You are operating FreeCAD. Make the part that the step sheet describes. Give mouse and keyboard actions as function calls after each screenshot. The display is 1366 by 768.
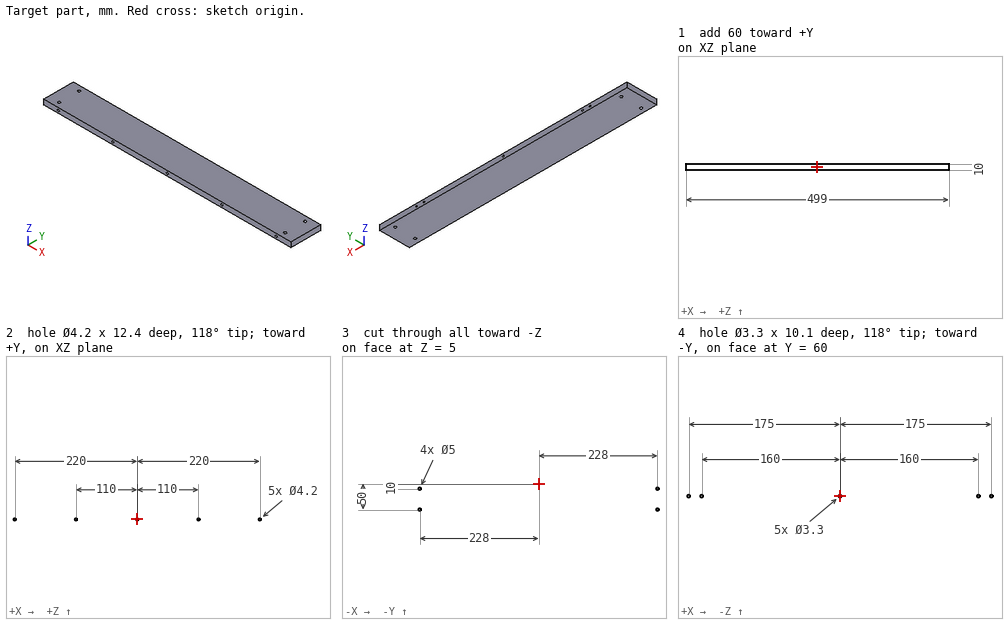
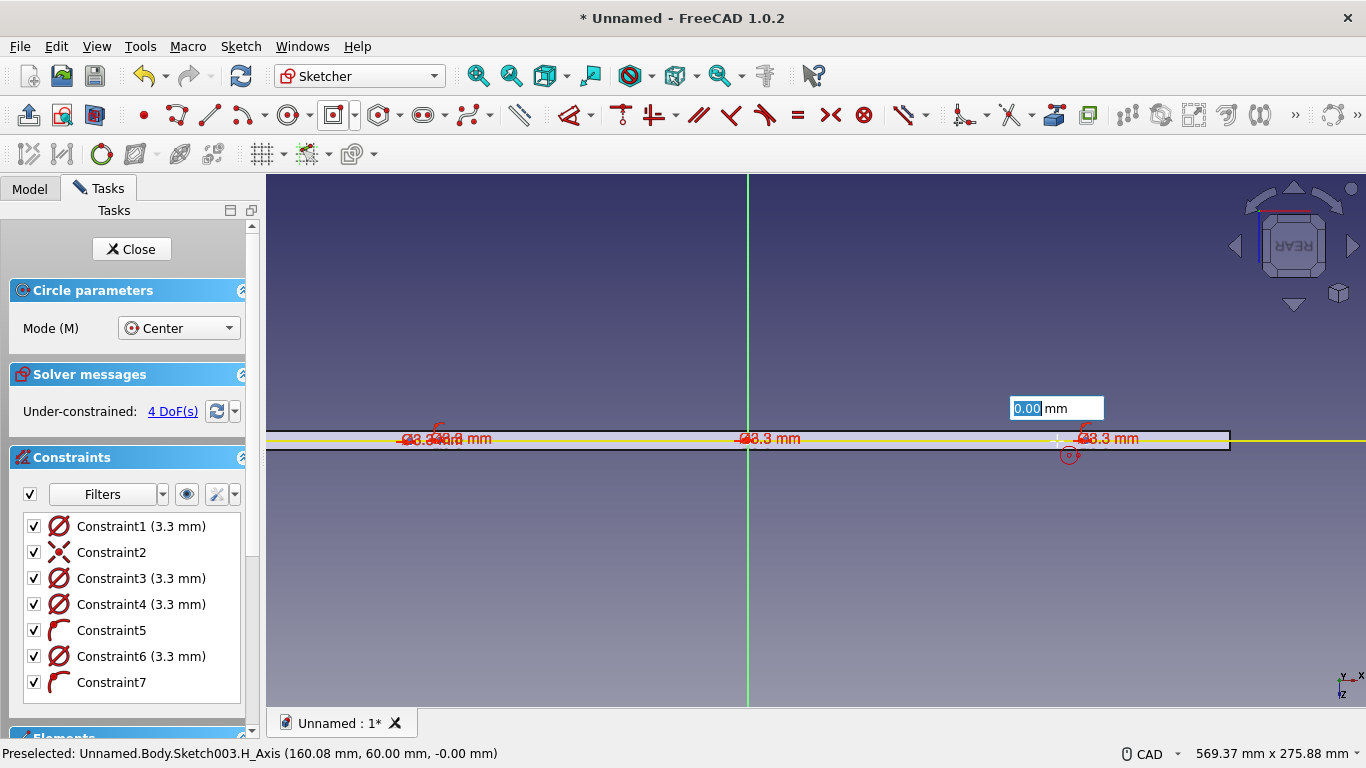
scroll(1056, 444, up, 9)
move(1051, 439)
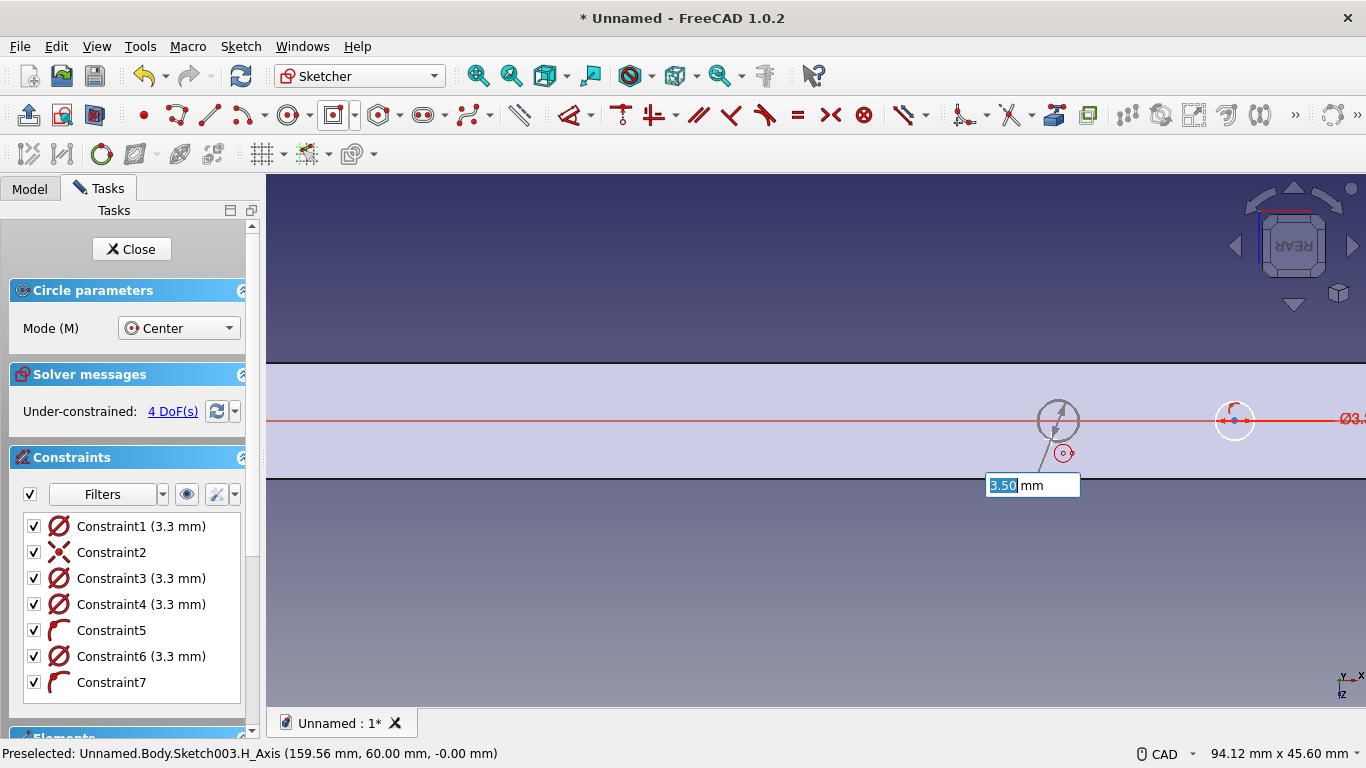
text(3.3)
key(Return)
key(Escape)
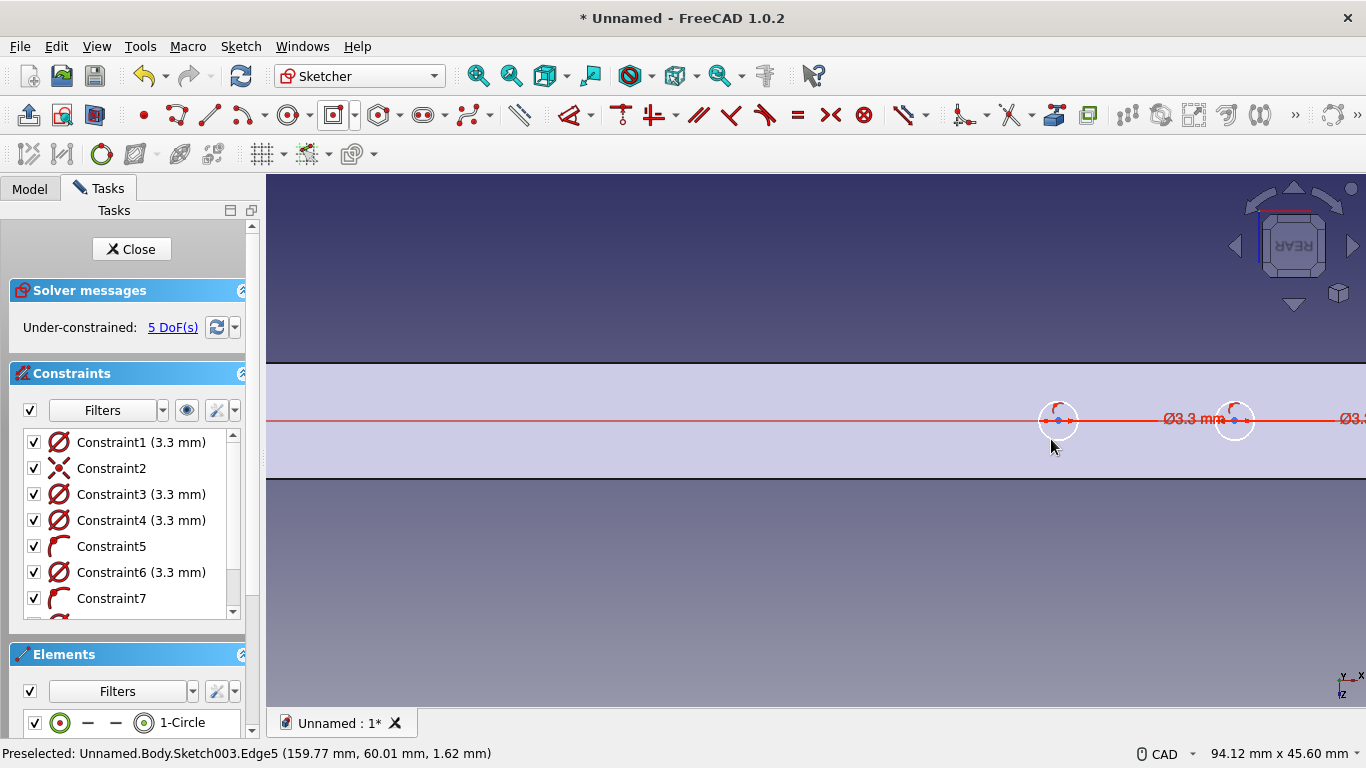
scroll(1056, 444, down, 9)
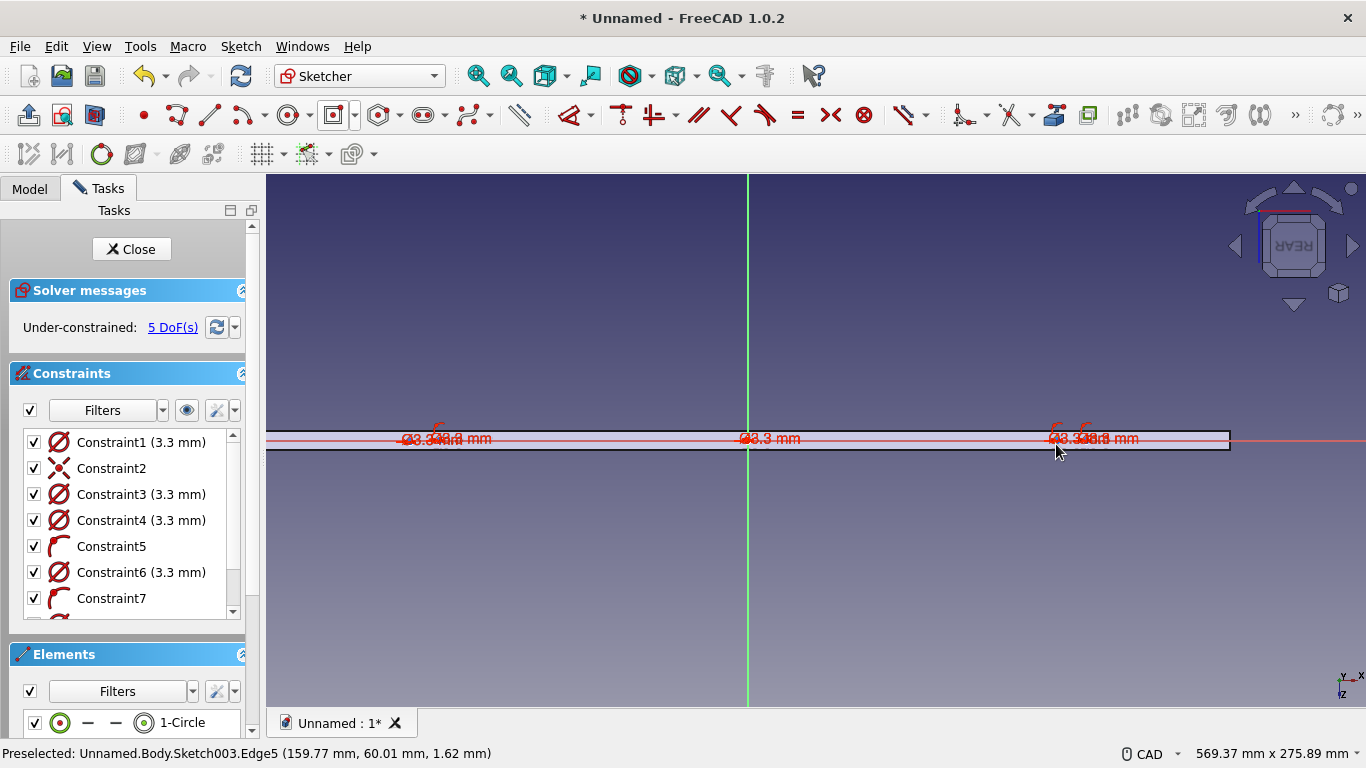
click(410, 442)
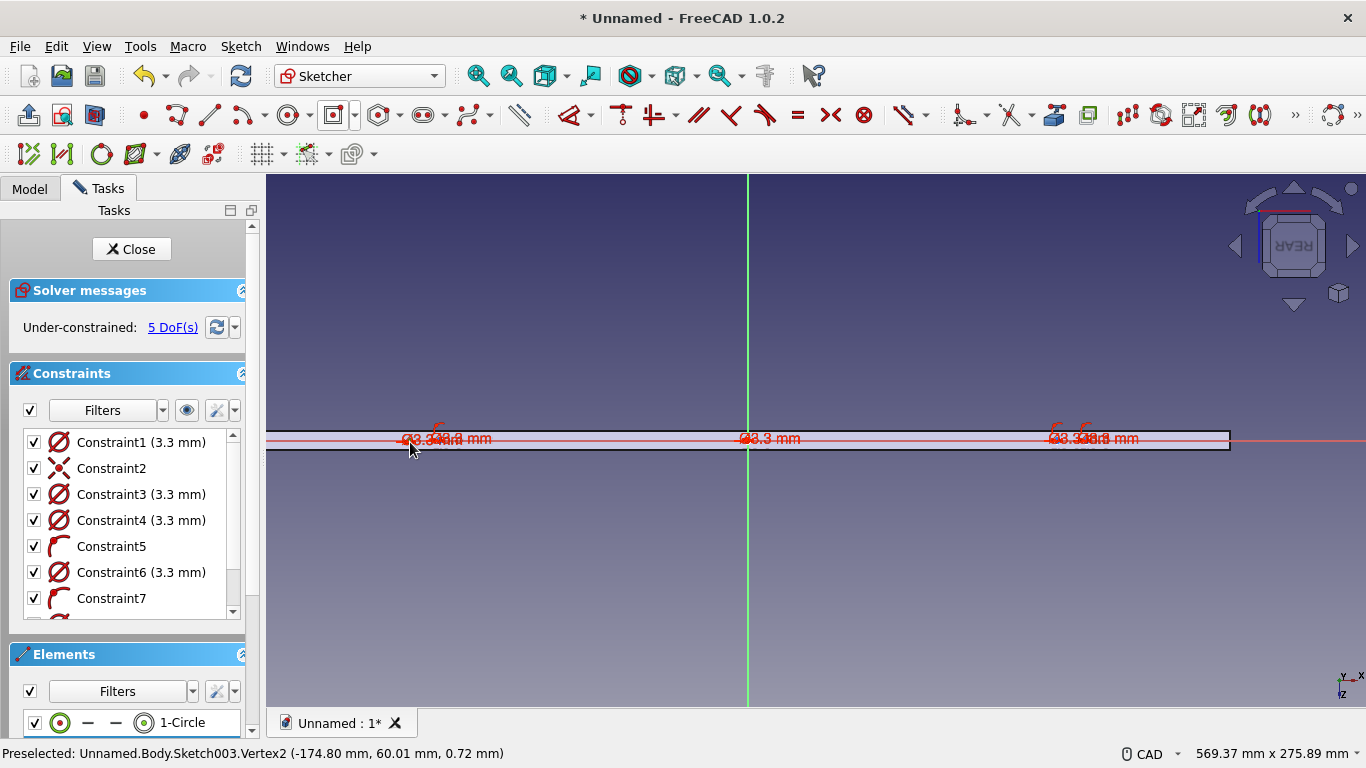
click(359, 441)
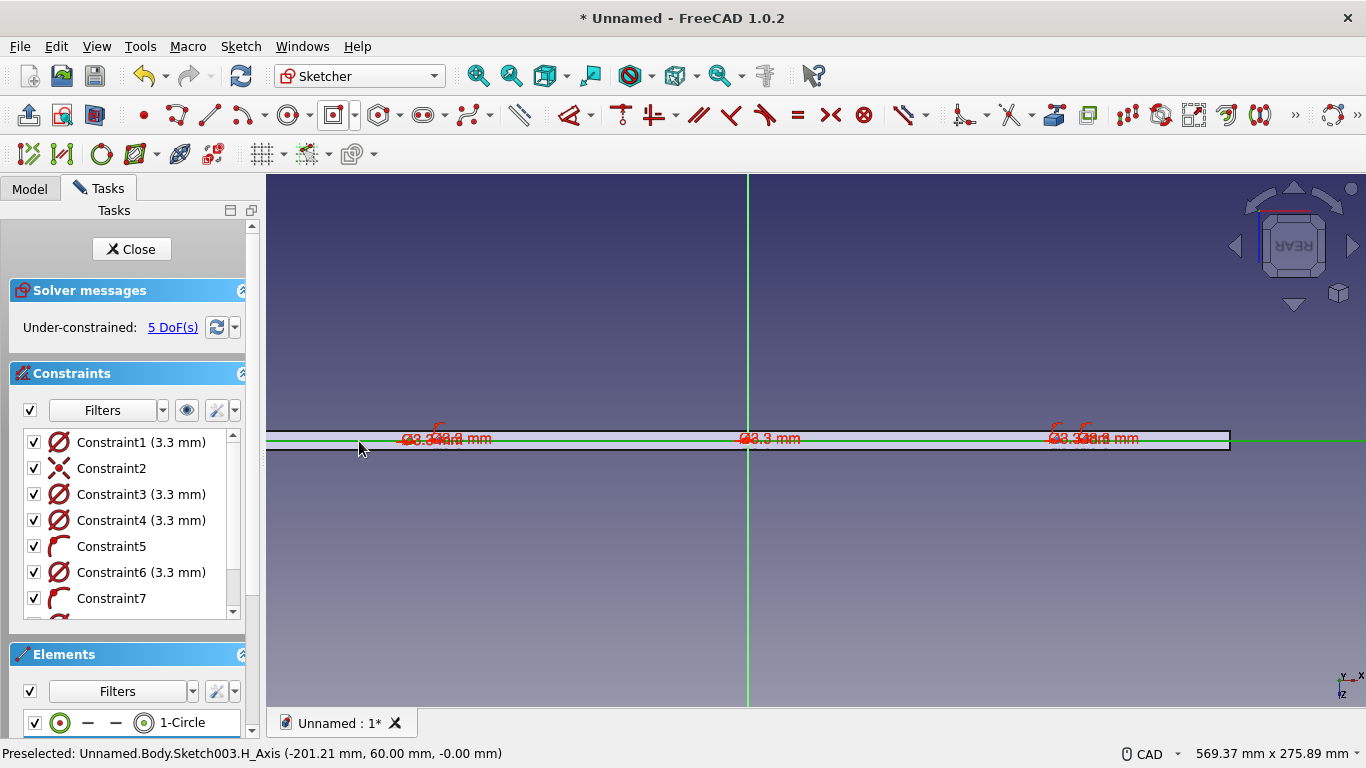
key(c)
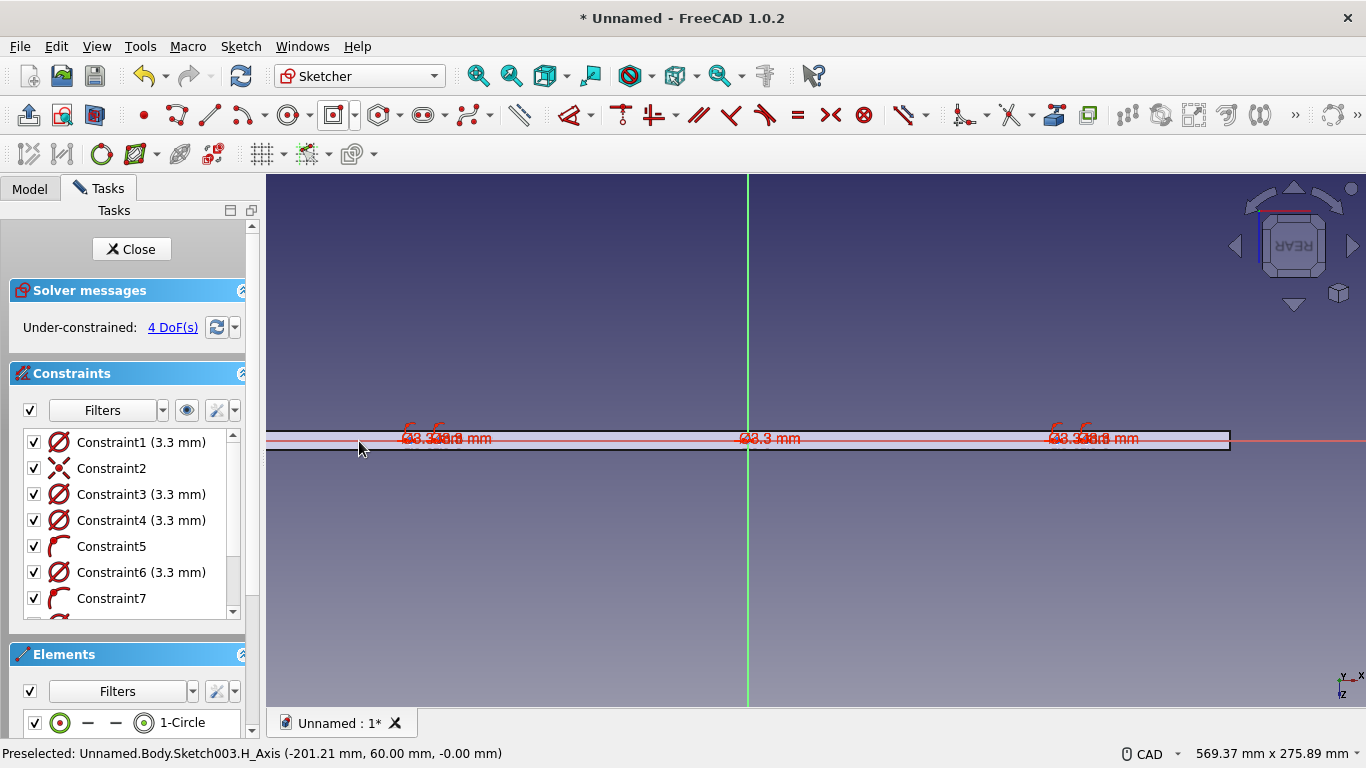
key(d)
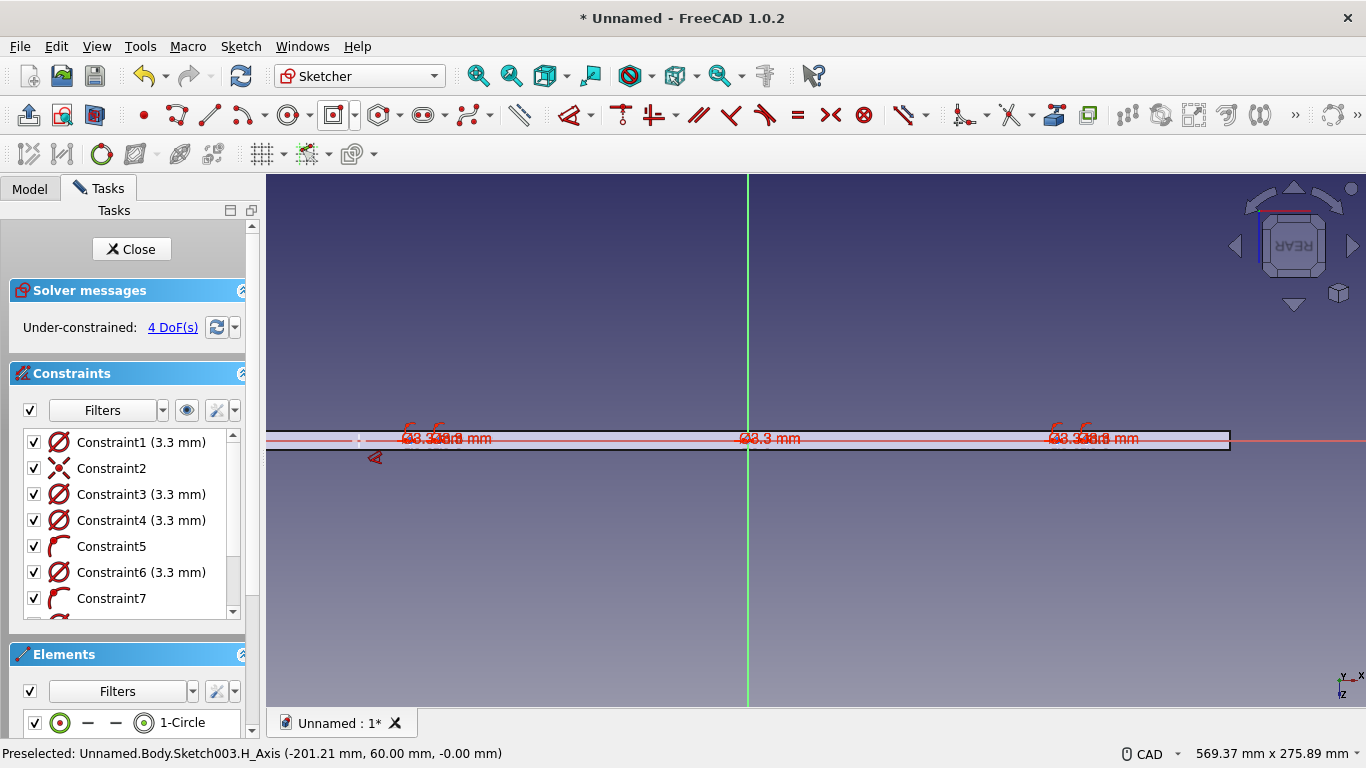
click(410, 441)
click(579, 475)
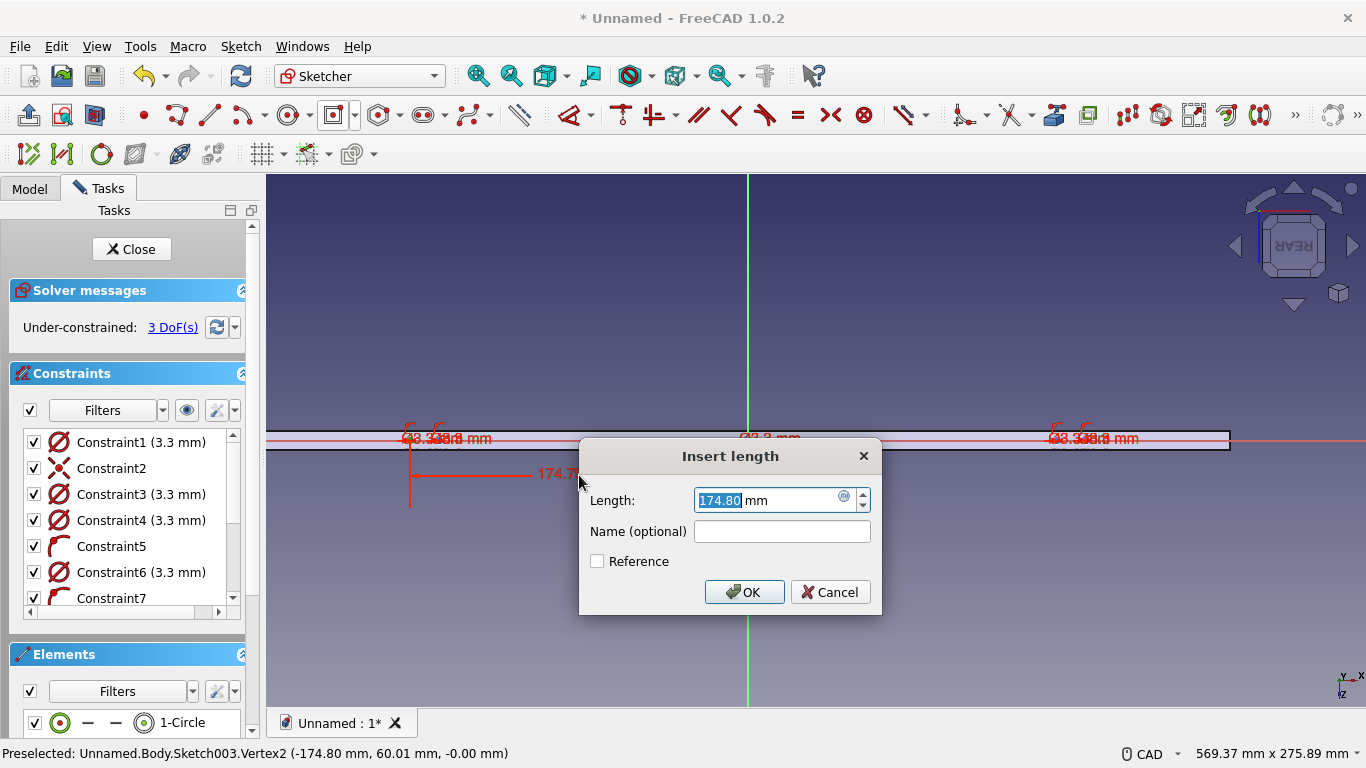
text(175)
key(Return)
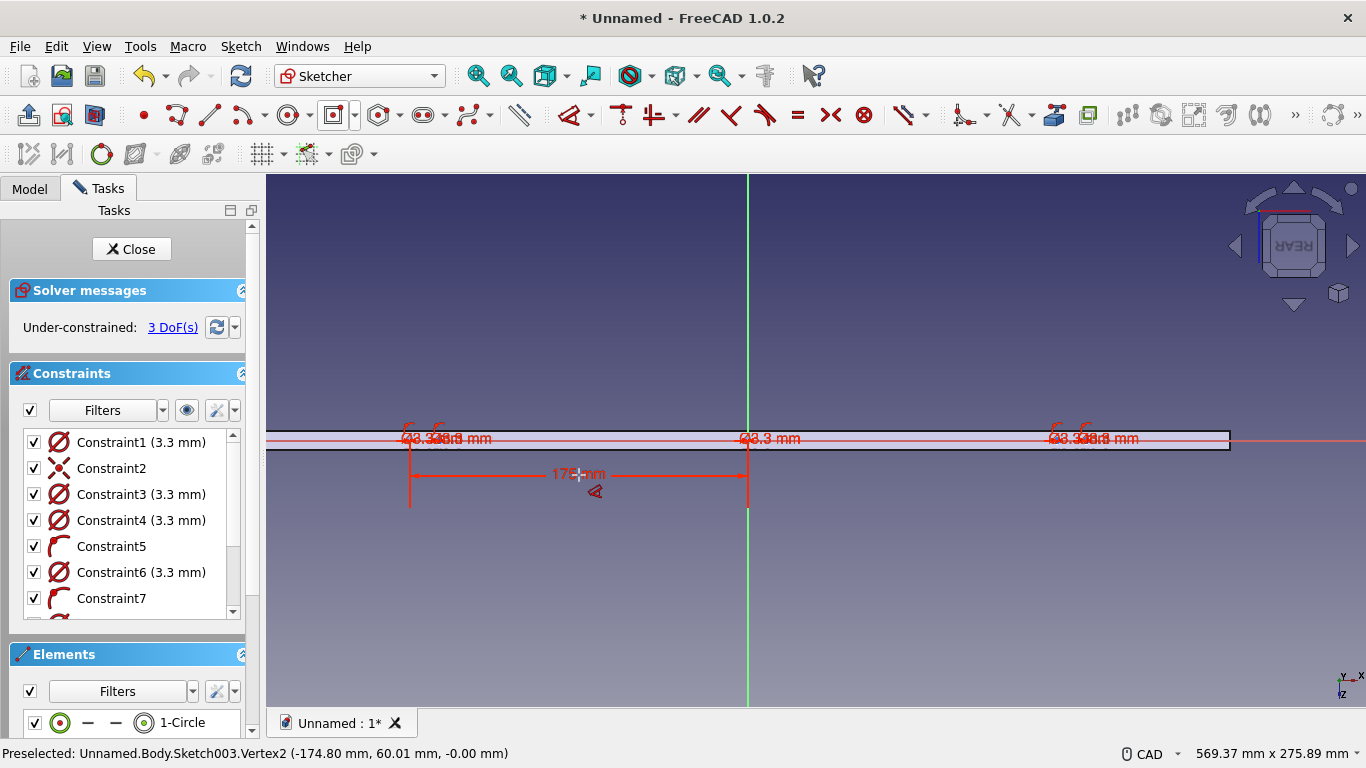
click(1086, 441)
click(917, 475)